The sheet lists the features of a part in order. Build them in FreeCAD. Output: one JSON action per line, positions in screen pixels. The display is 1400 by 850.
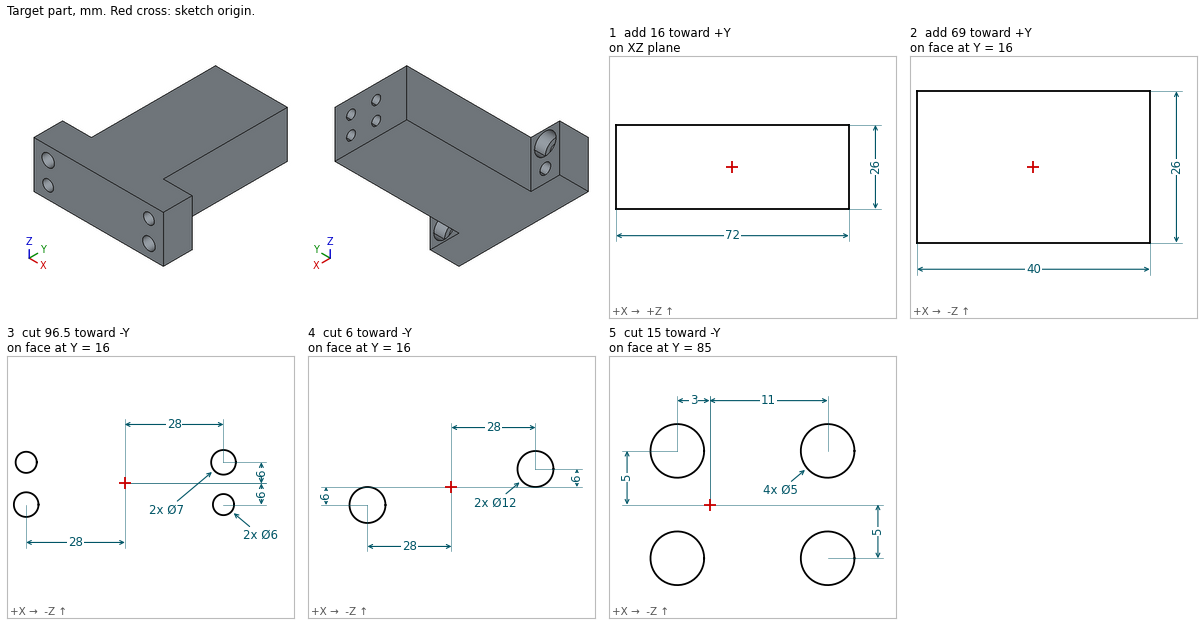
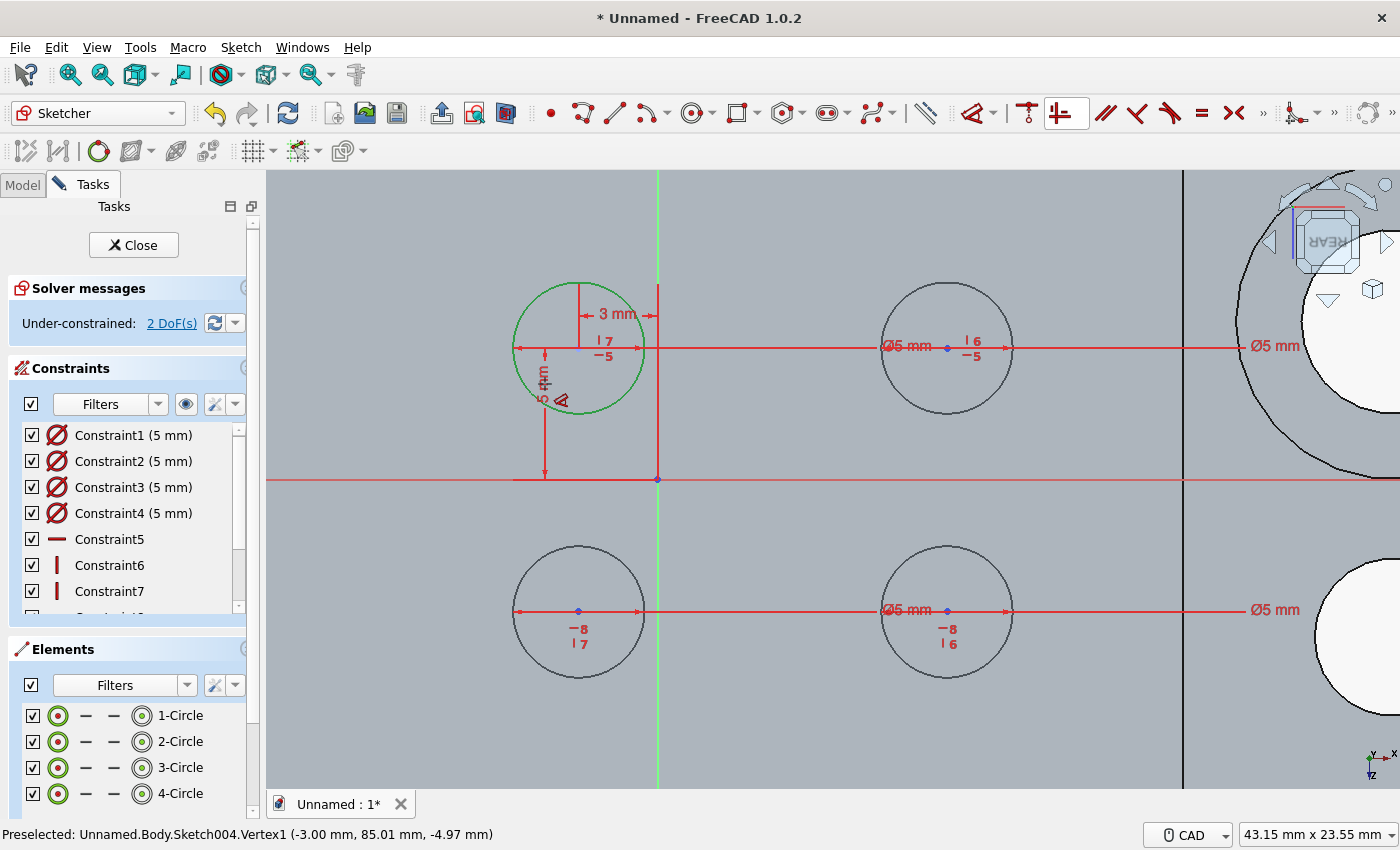
{"action": "left_click", "coordinate": [947, 612]}
{"action": "left_click", "coordinate": [981, 515]}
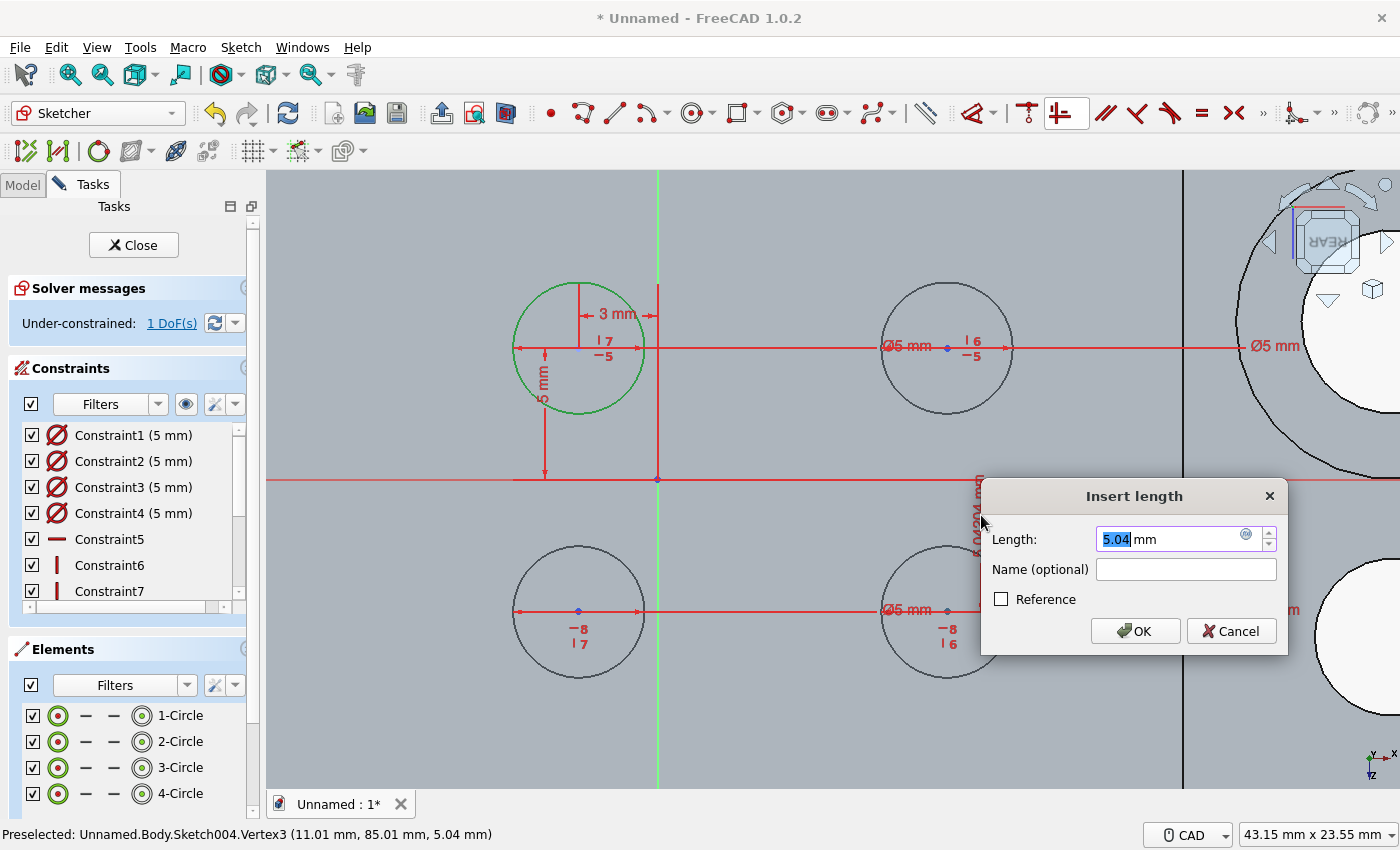
{"action": "type", "text": "5"}
{"action": "key", "text": "Return"}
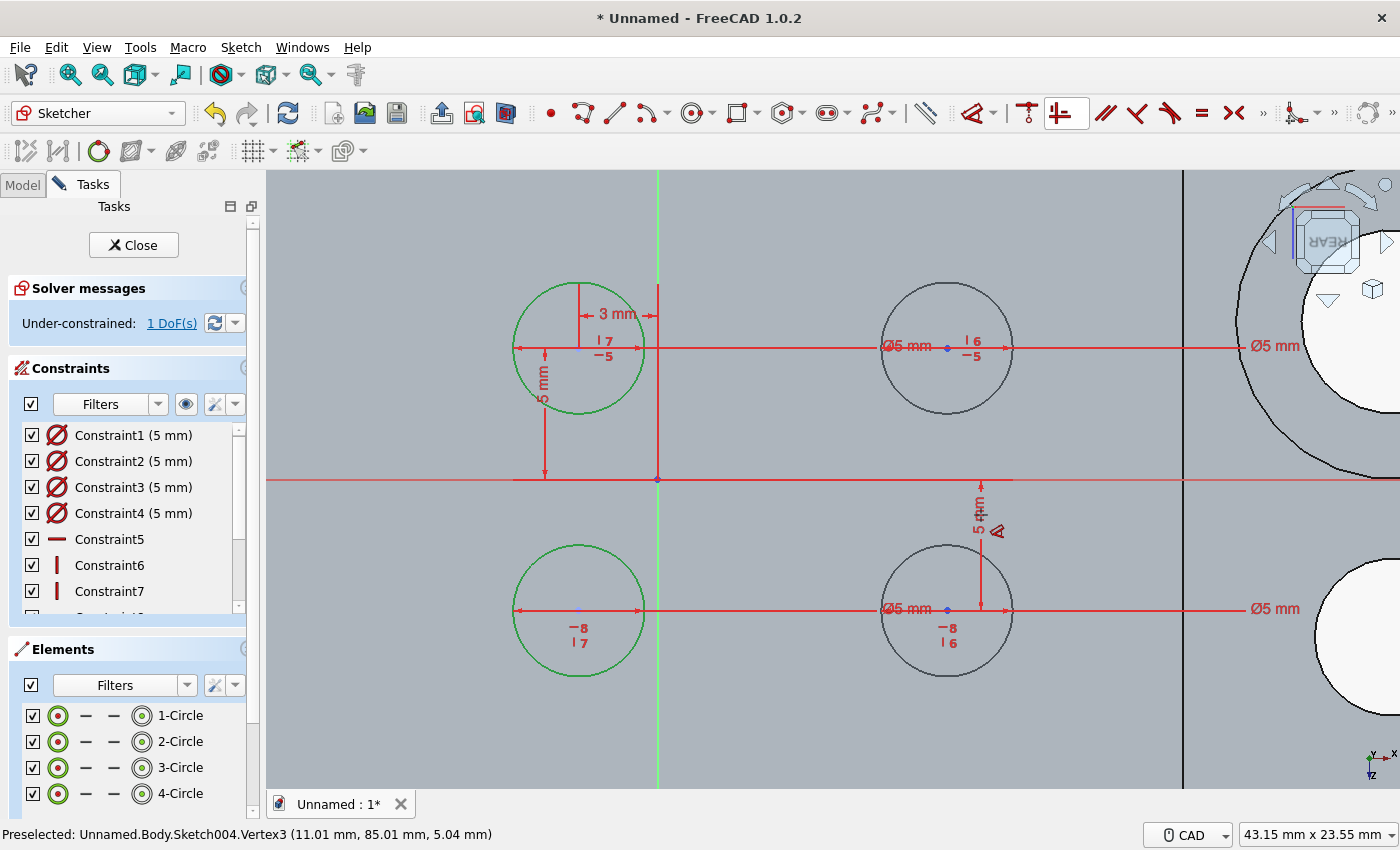
{"action": "left_click", "coordinate": [947, 348]}
{"action": "left_click", "coordinate": [802, 314]}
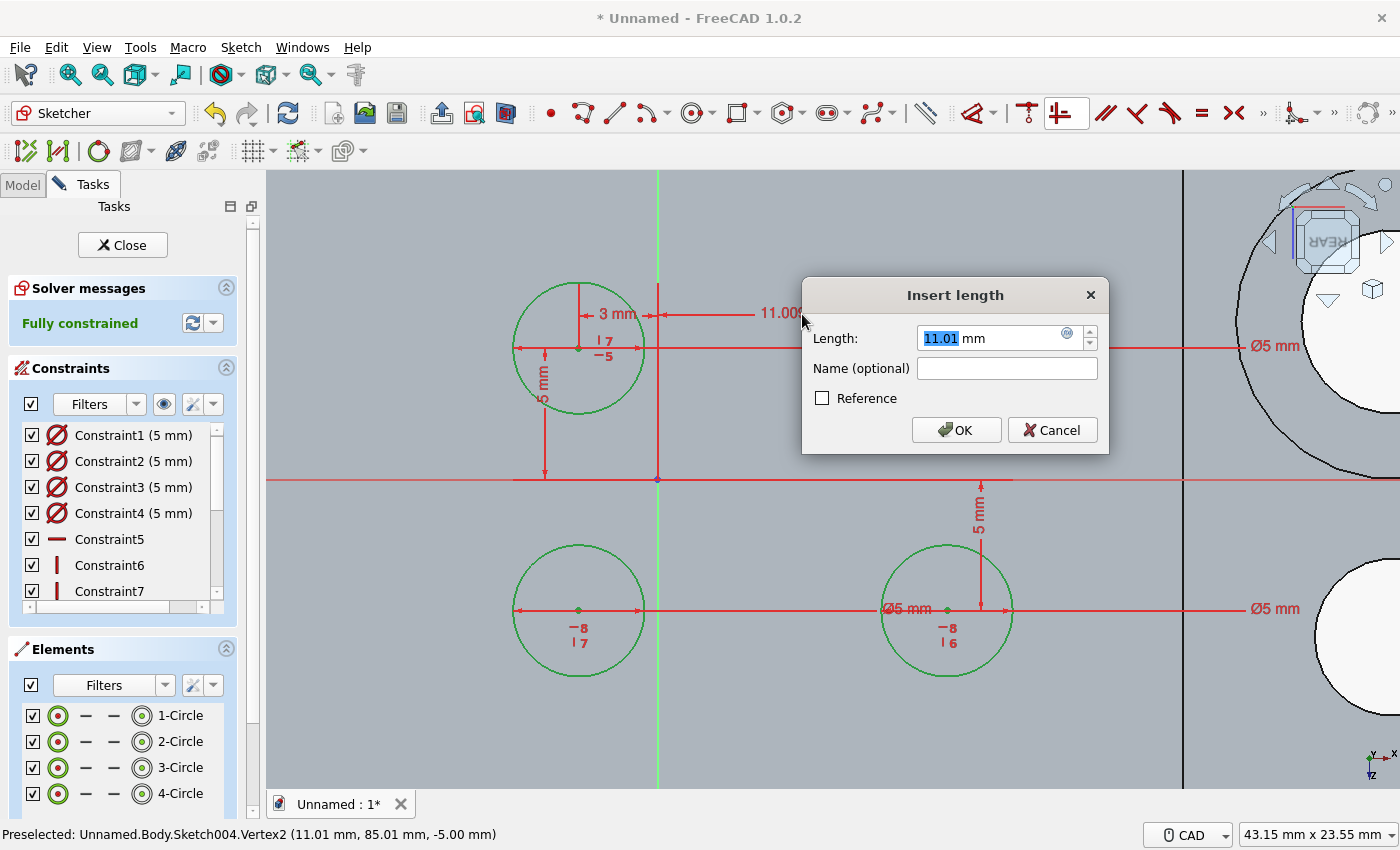
{"action": "type", "text": "11"}
{"action": "key", "text": "Return"}
{"action": "key", "text": "Escape"}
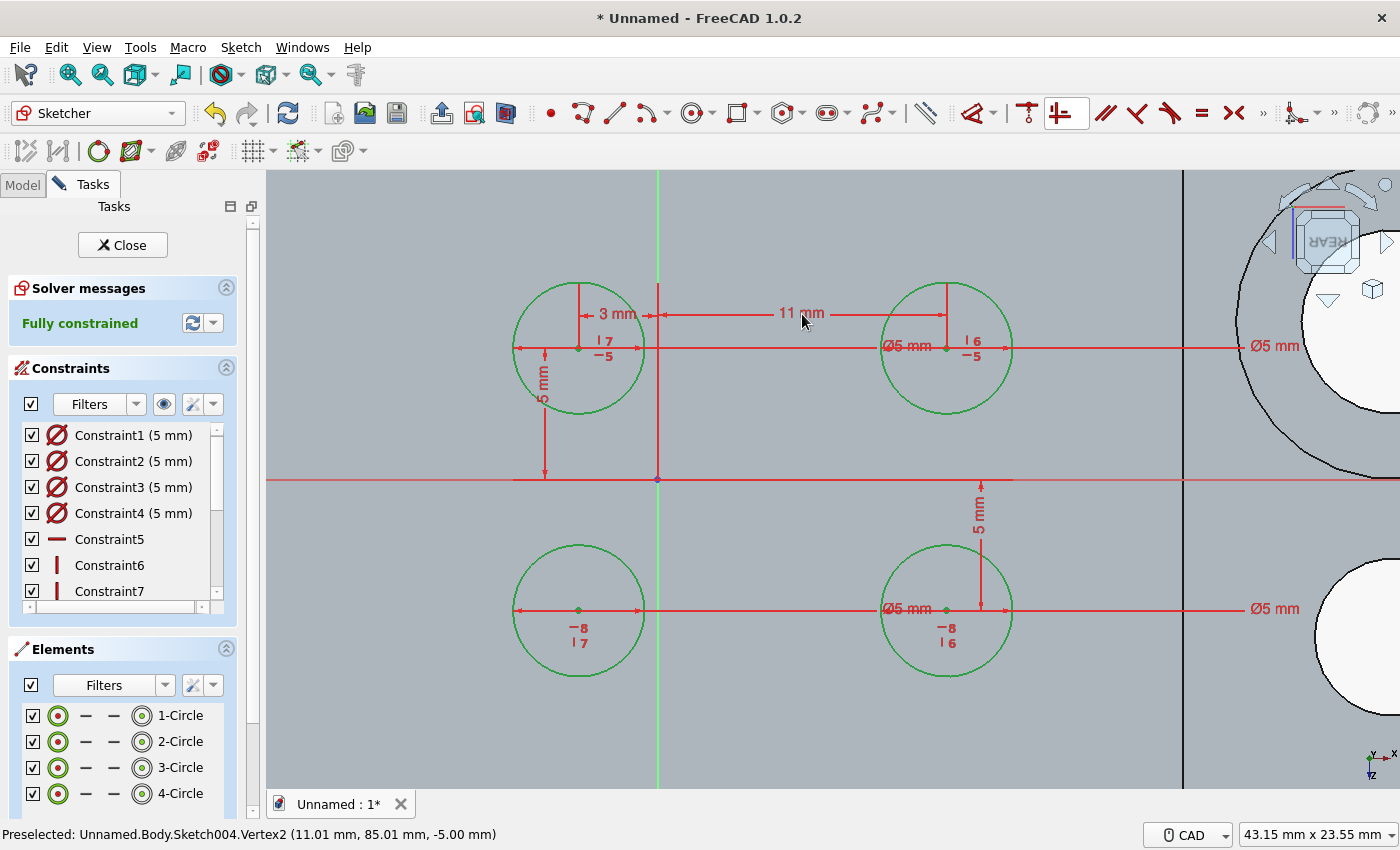
{"action": "left_click", "coordinate": [123, 245]}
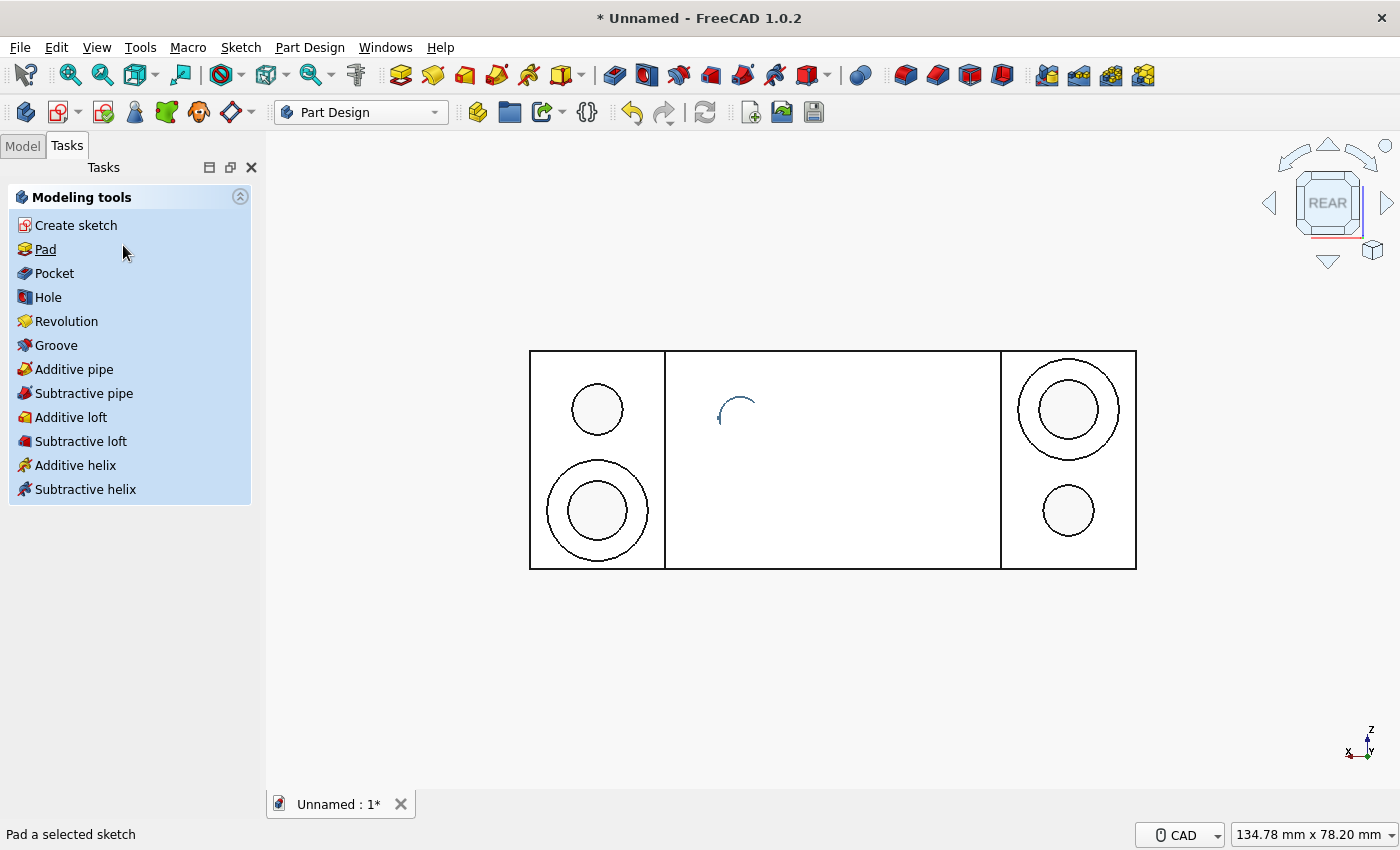
{"action": "left_click", "coordinate": [616, 76]}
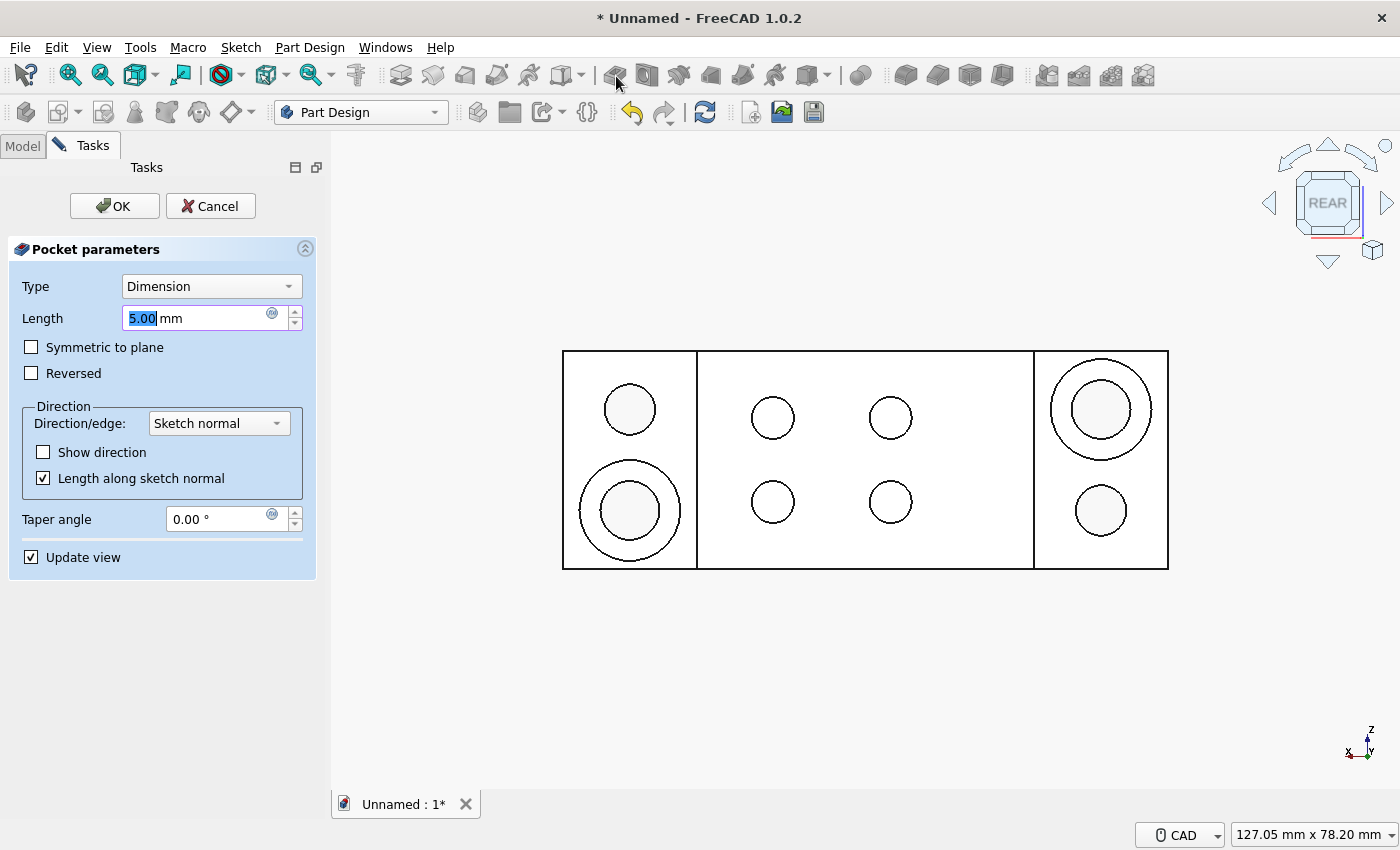
{"action": "type", "text": "15"}
{"action": "key", "text": "Tab"}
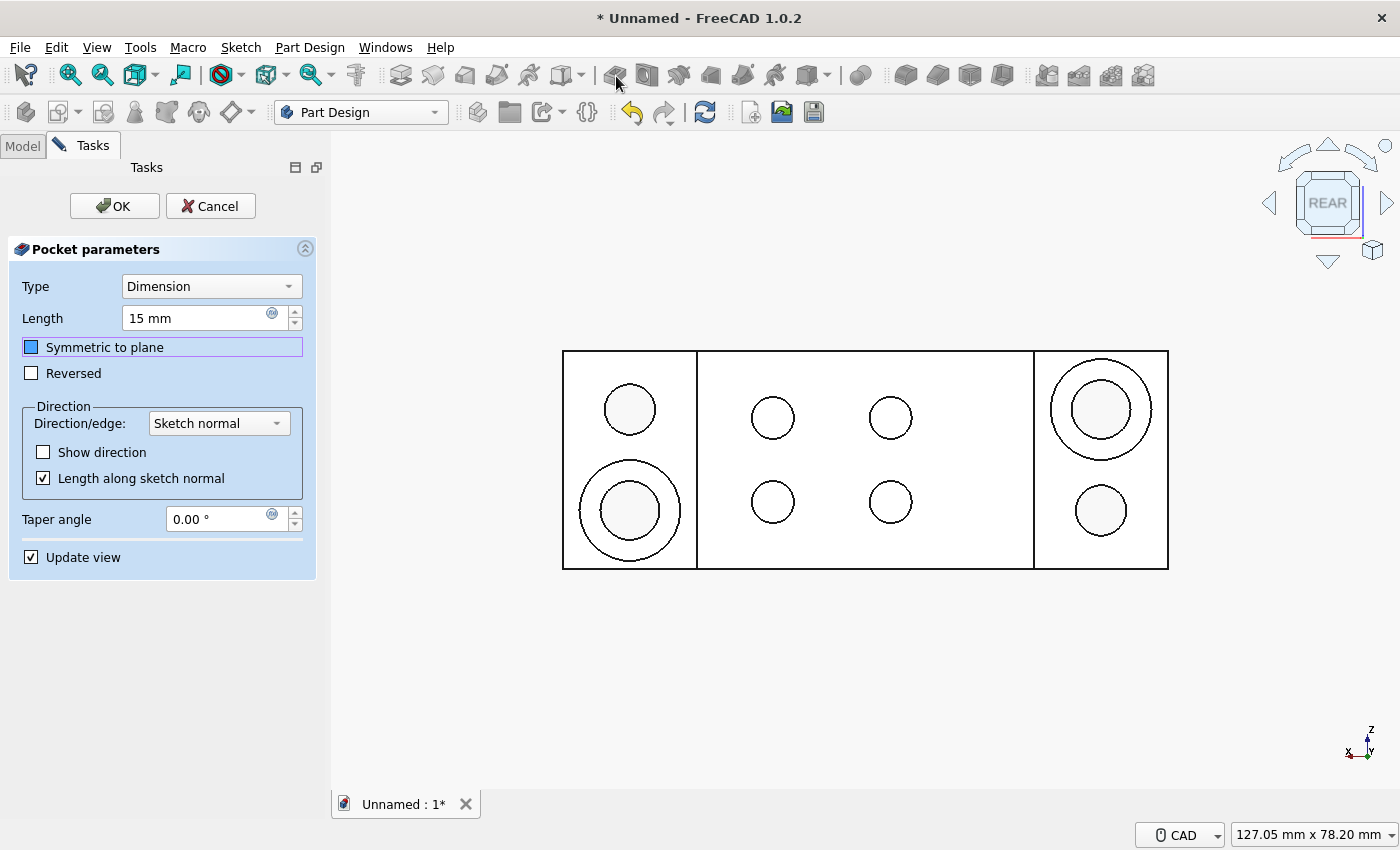
{"action": "left_click", "coordinate": [115, 206]}